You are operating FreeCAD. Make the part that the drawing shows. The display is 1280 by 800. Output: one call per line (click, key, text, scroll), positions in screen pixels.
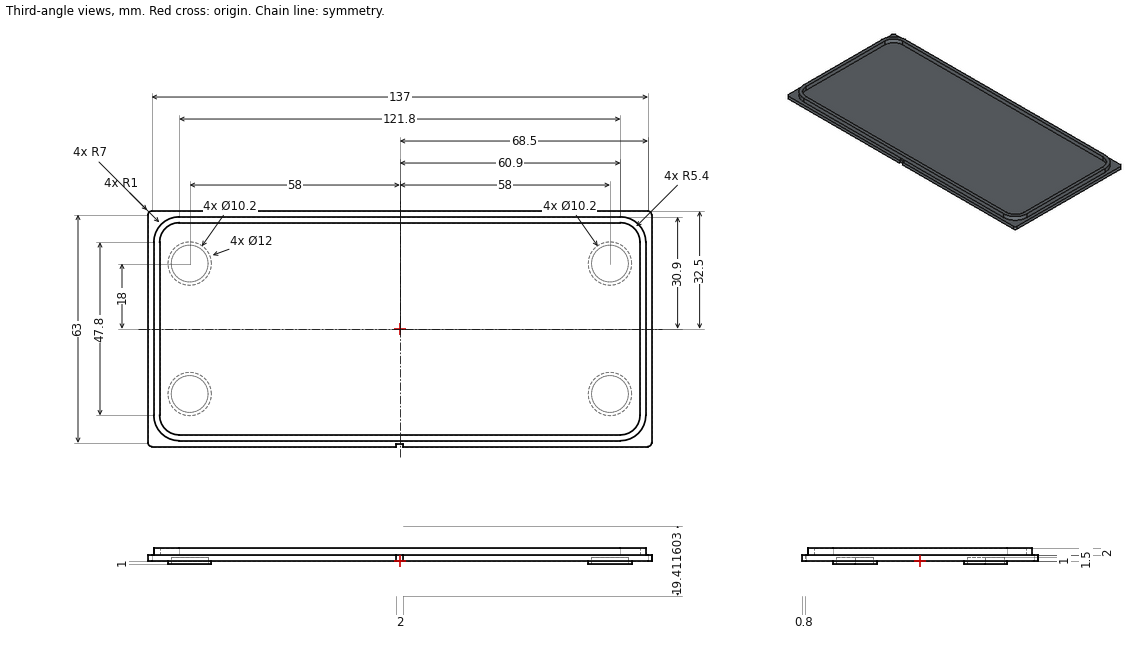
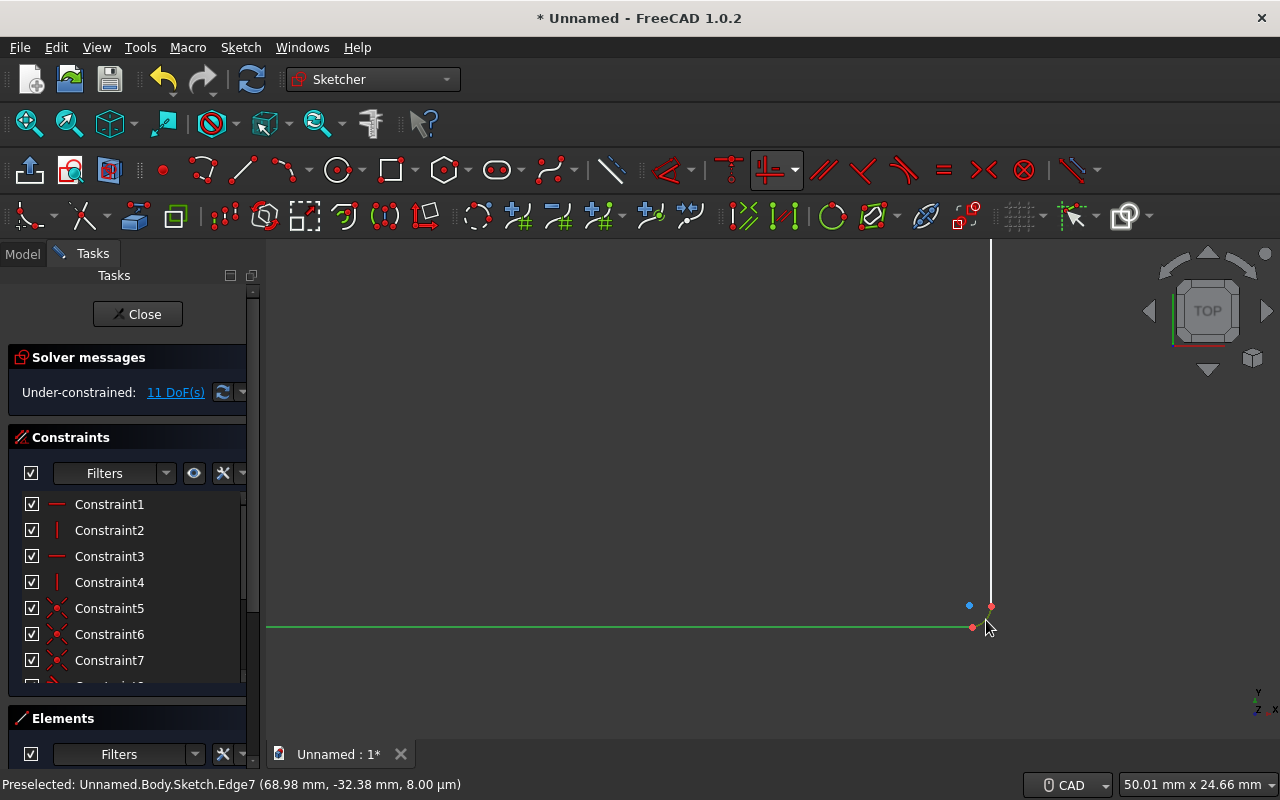
click(904, 170)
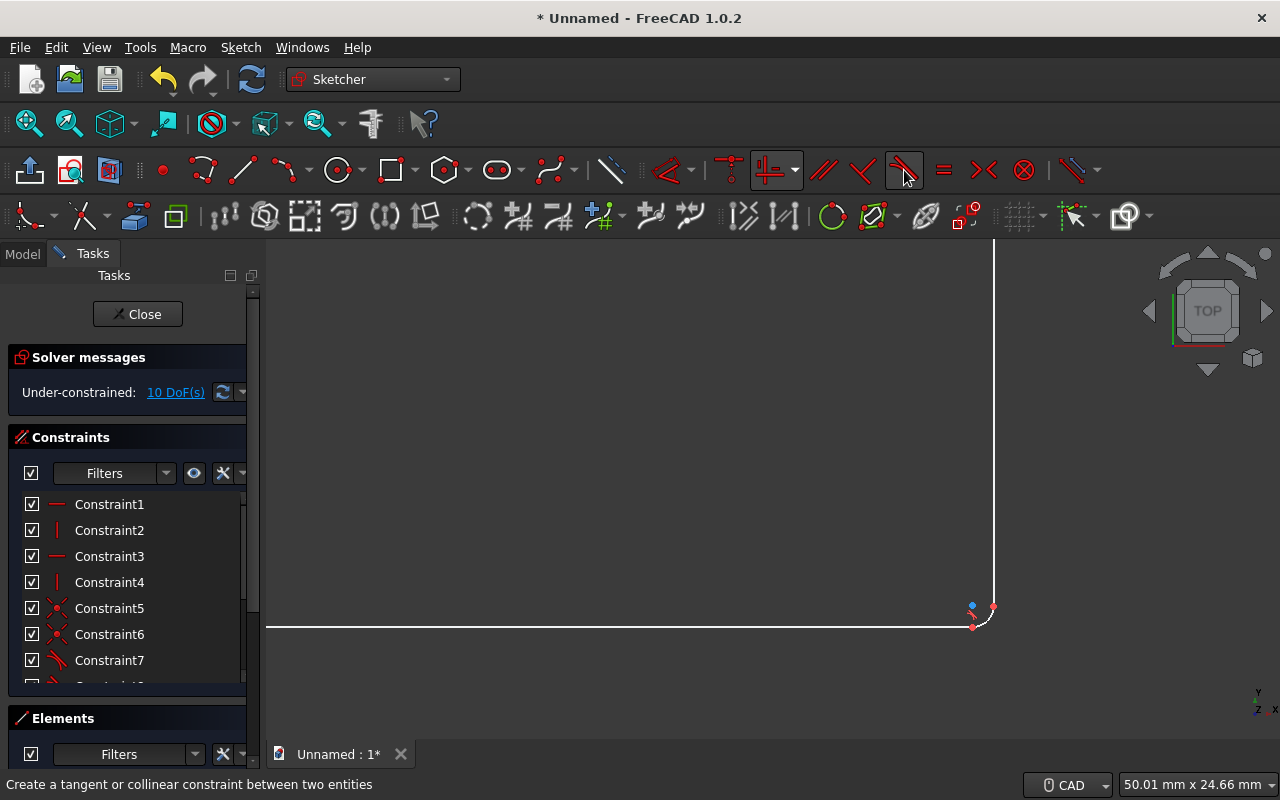
scroll(988, 621, down, 8)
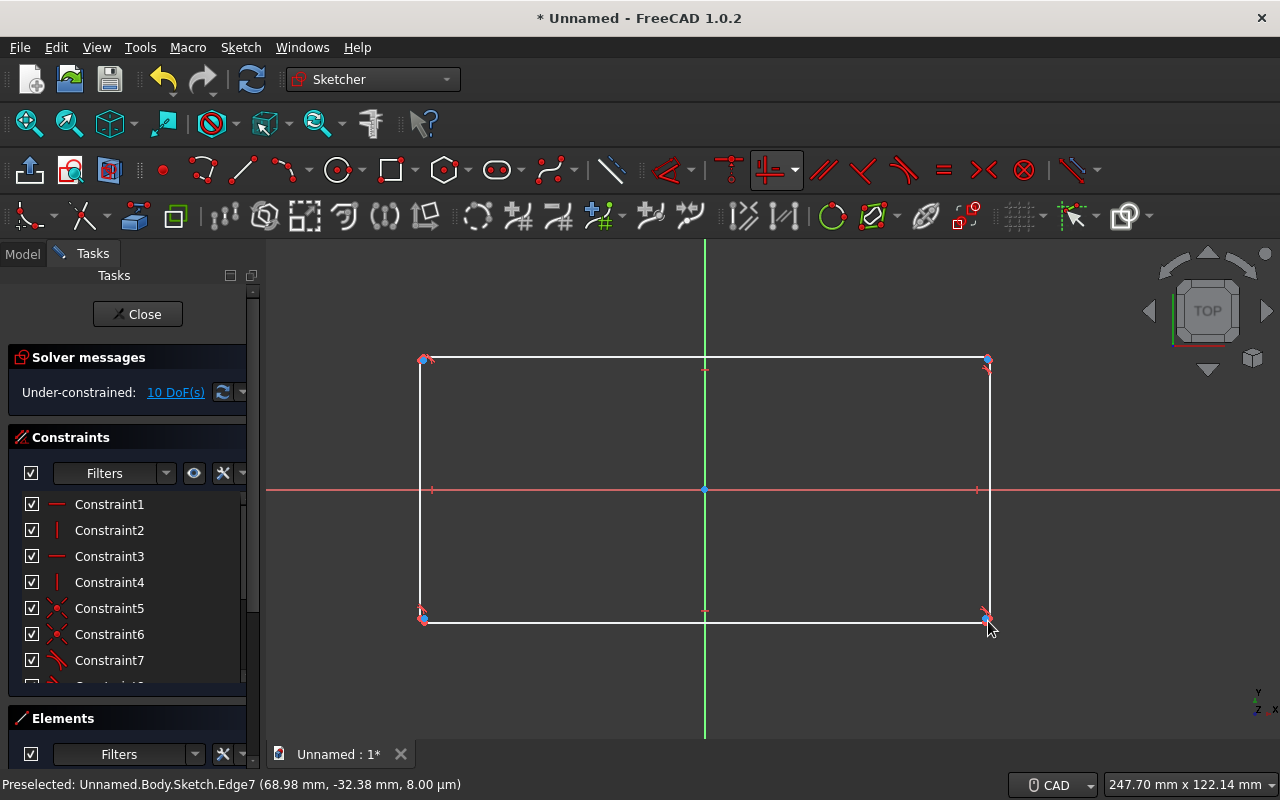
click(990, 567)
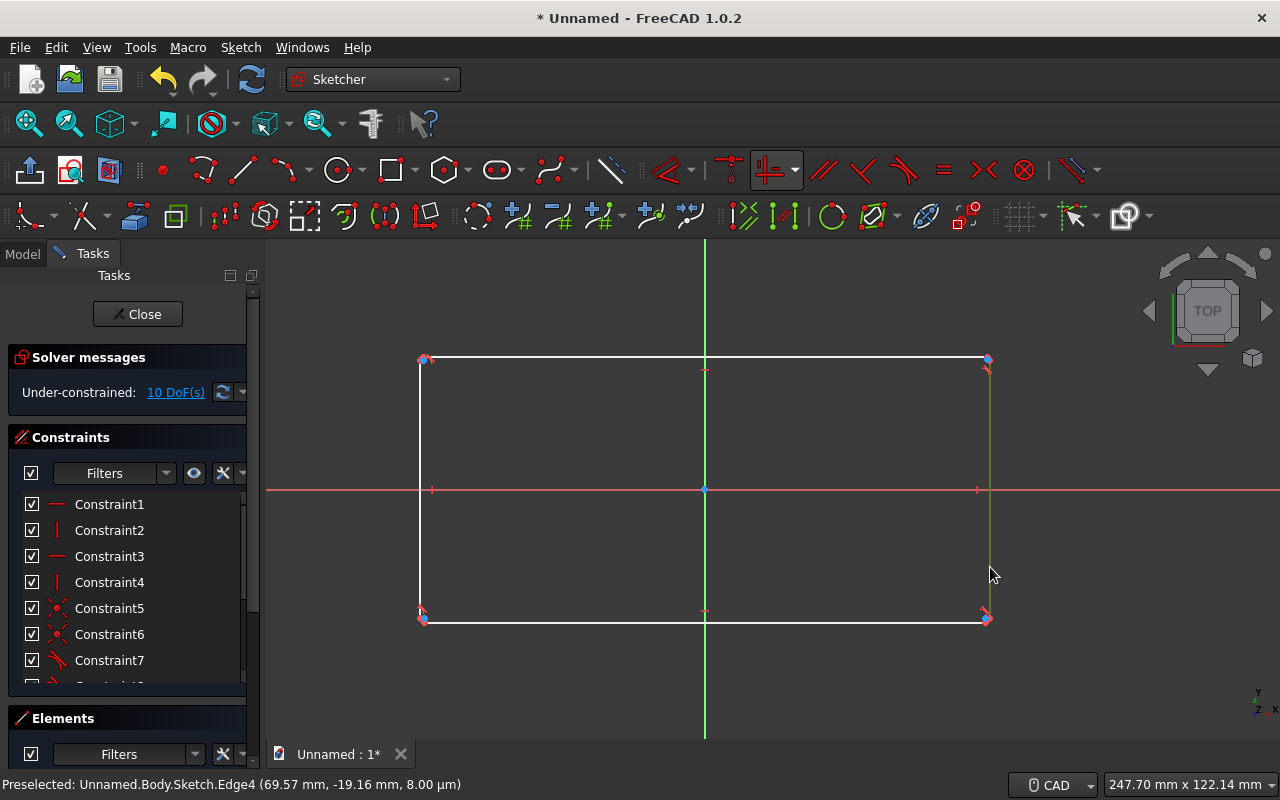
scroll(988, 622, up, 8)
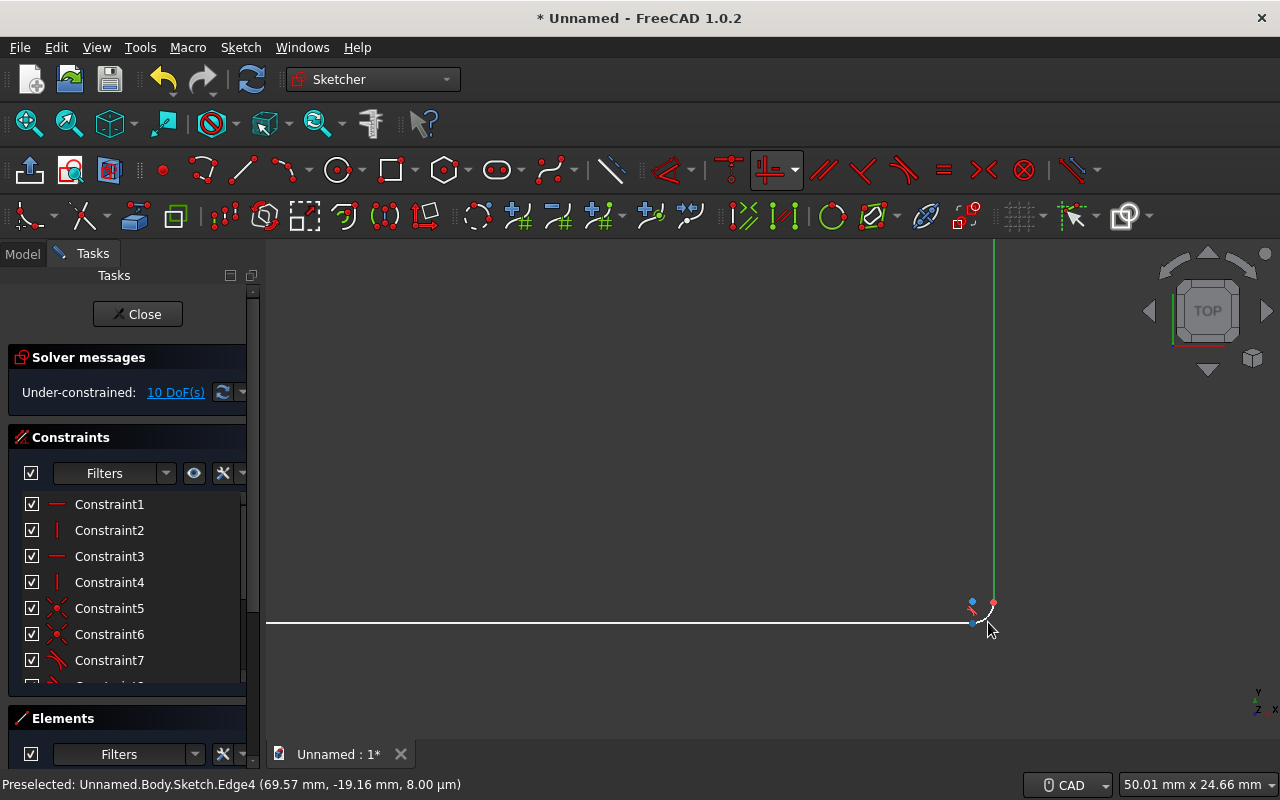
click(987, 617)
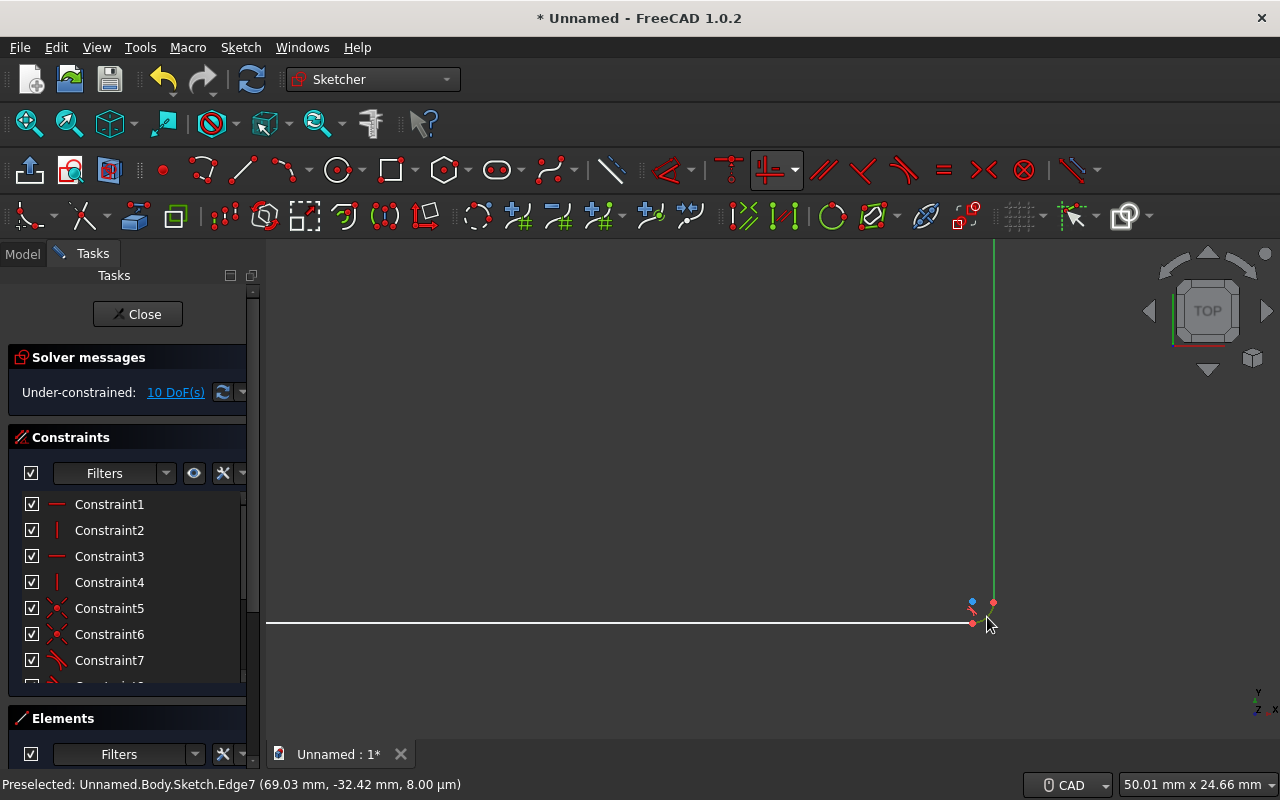
click(904, 170)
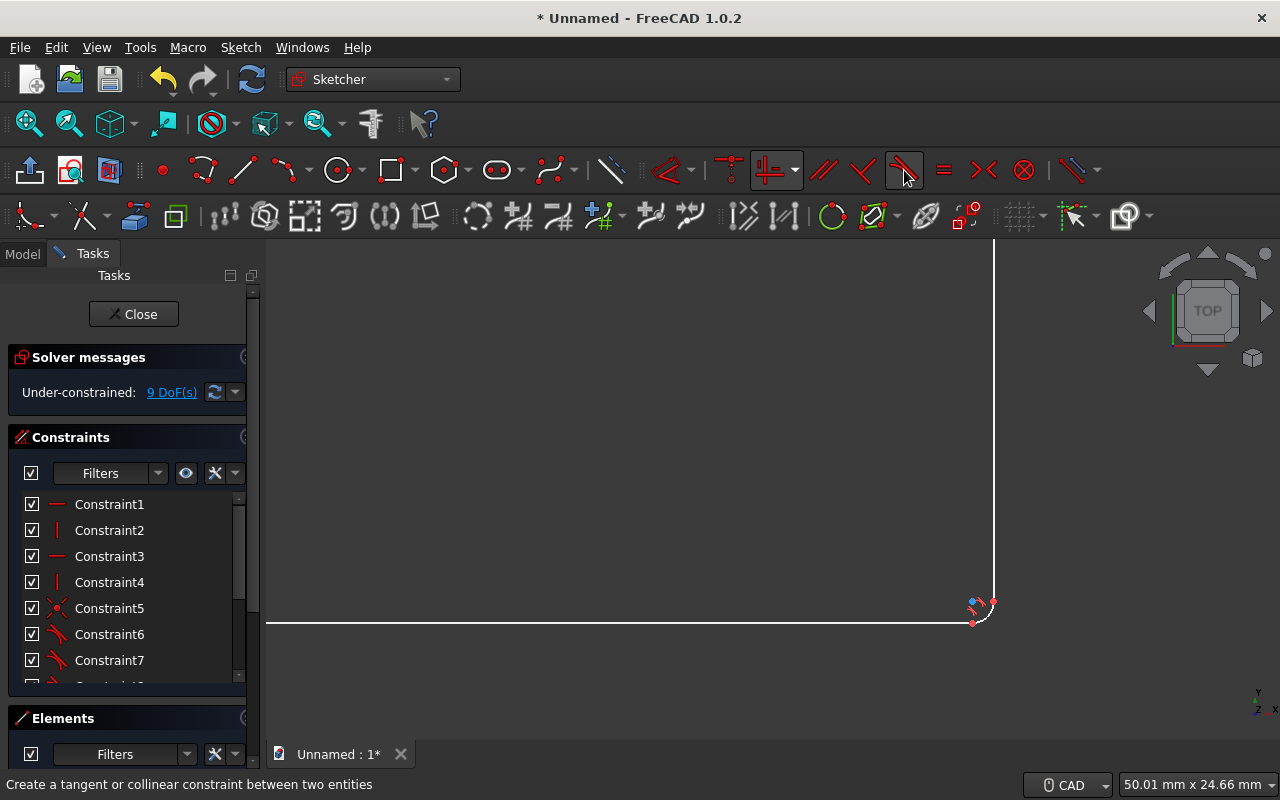
scroll(988, 622, down, 8)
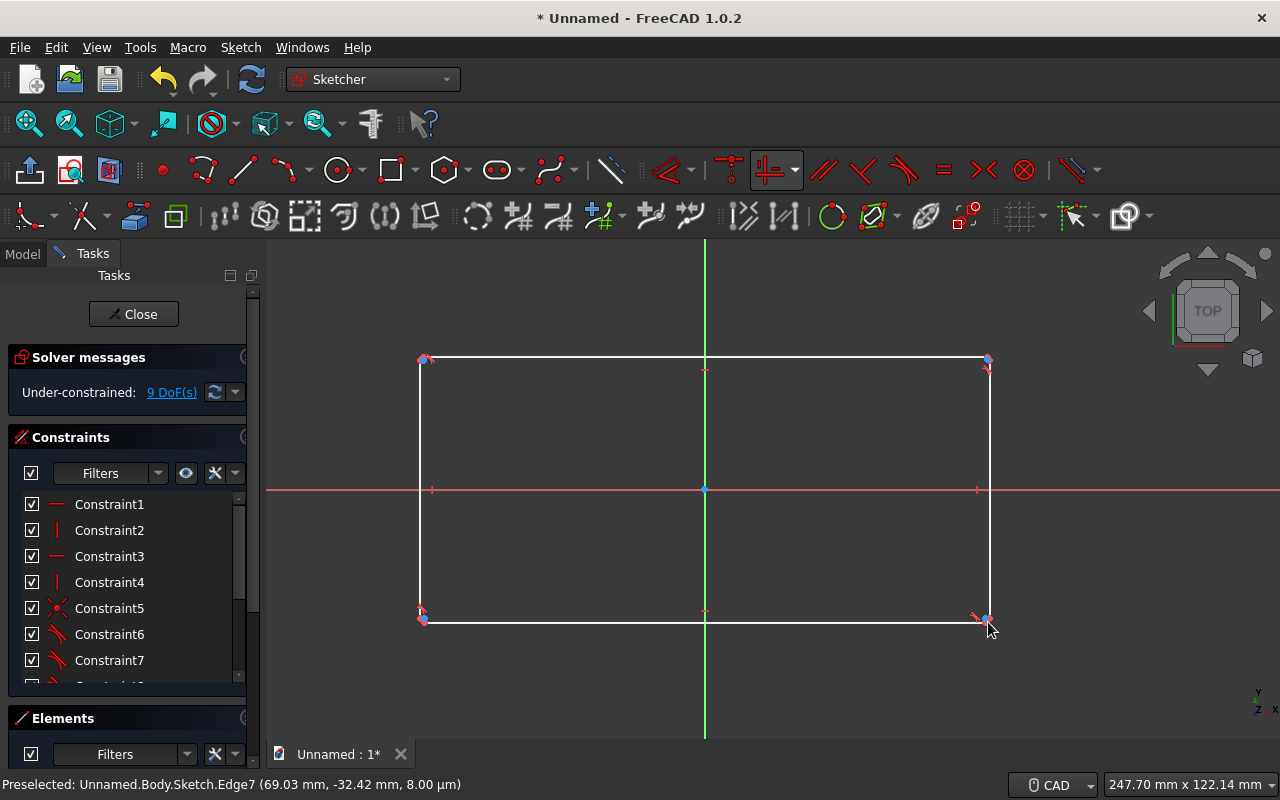
click(990, 567)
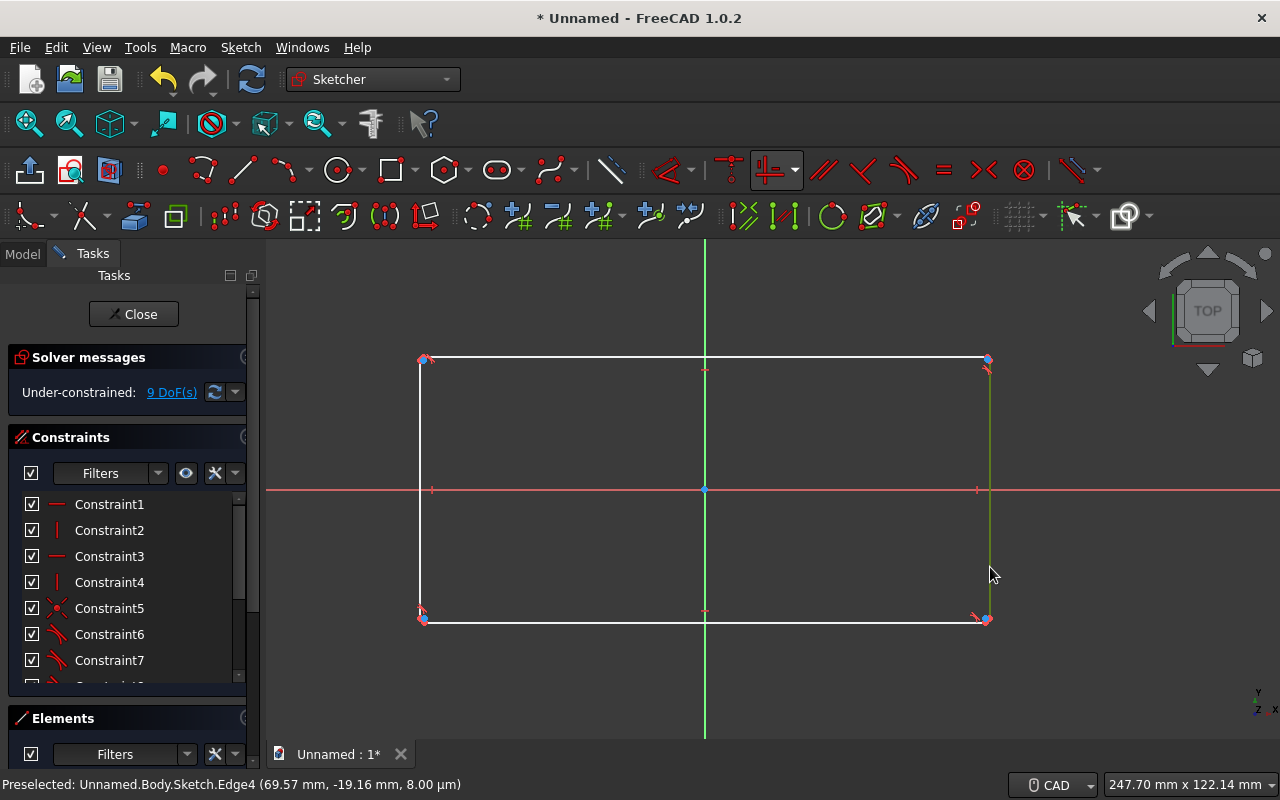
scroll(989, 358, up, 9)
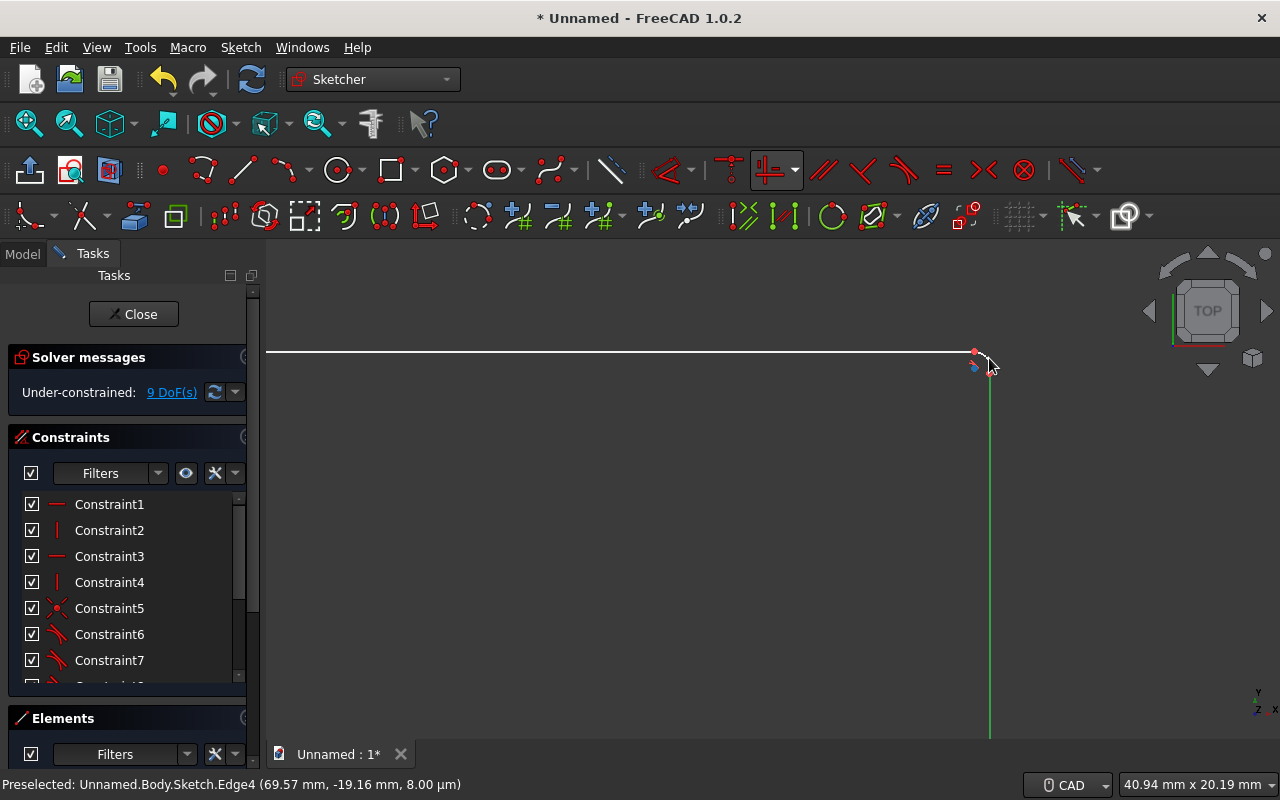
click(987, 359)